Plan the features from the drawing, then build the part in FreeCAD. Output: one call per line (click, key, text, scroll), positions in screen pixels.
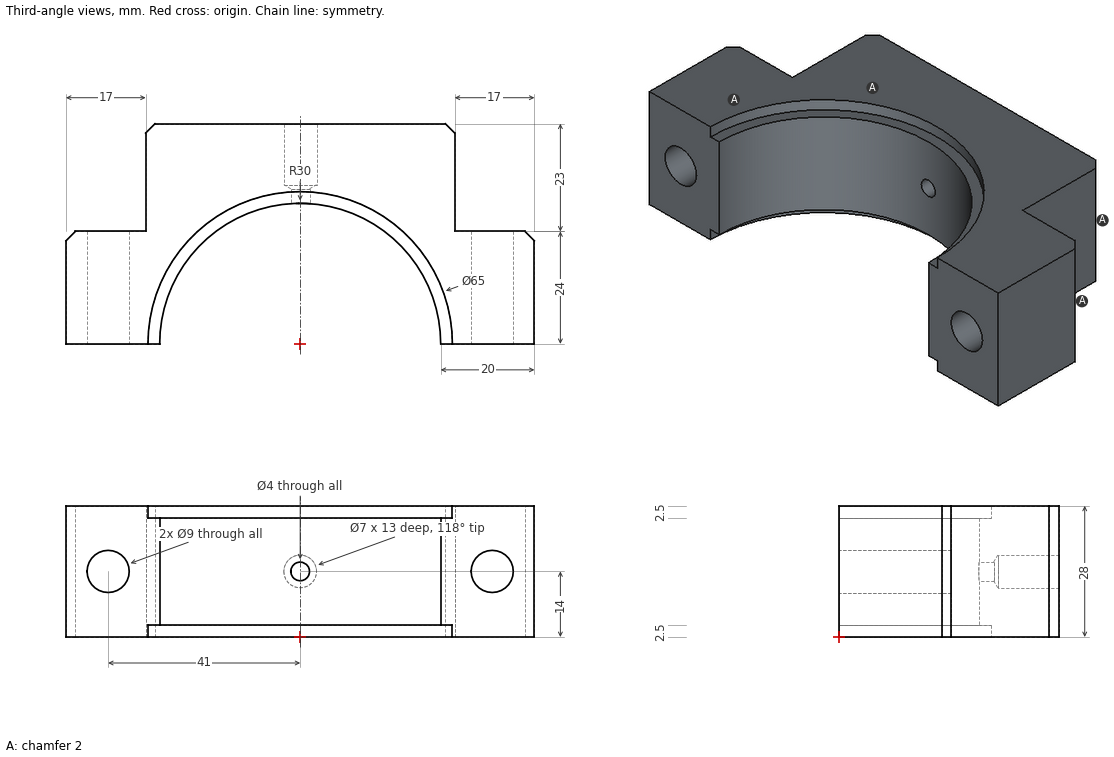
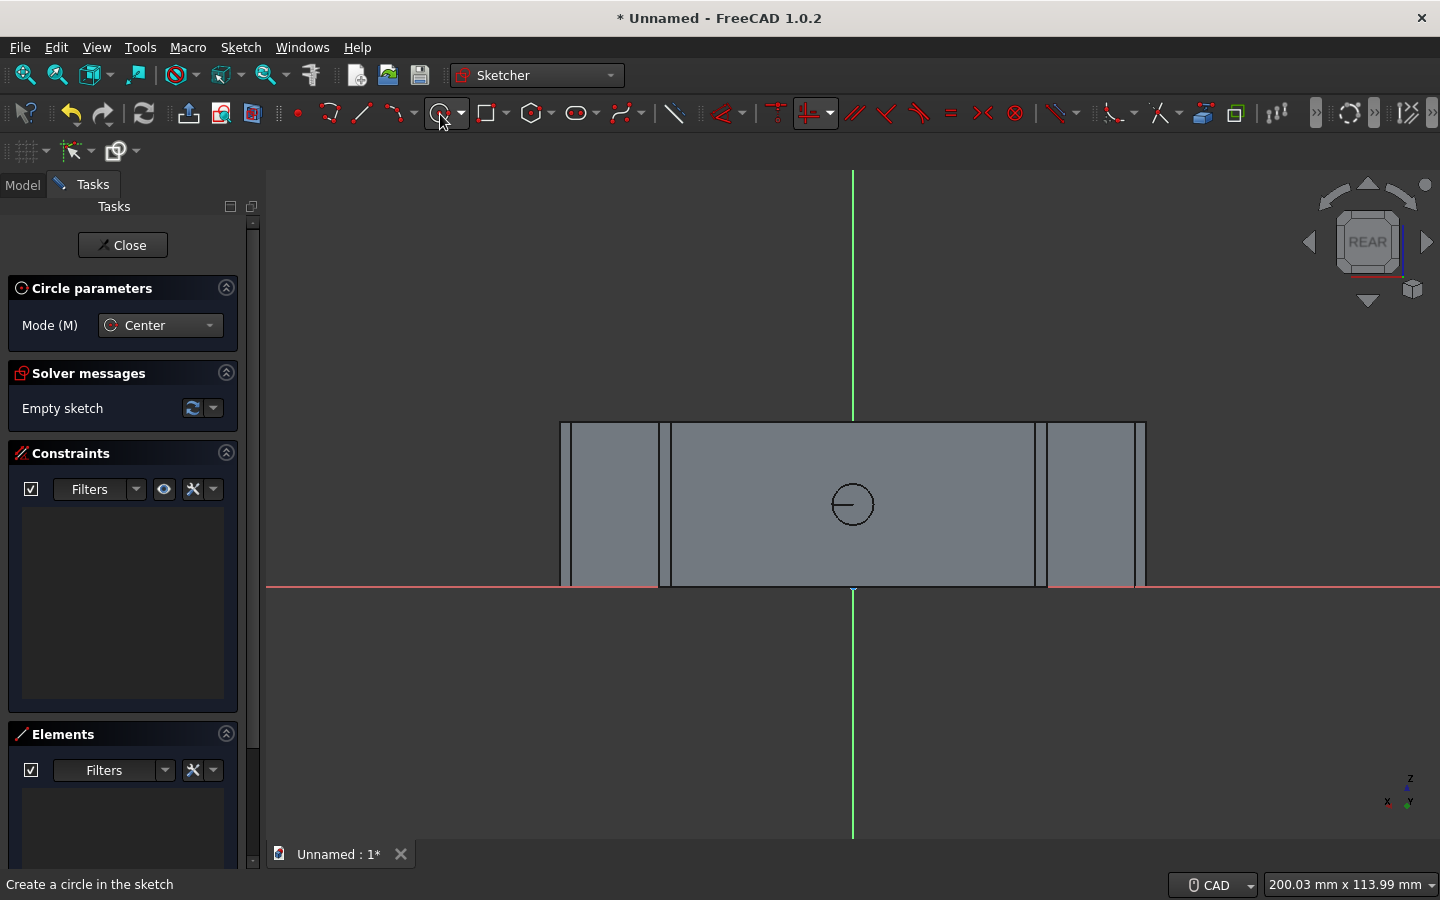
click(1094, 505)
click(1112, 486)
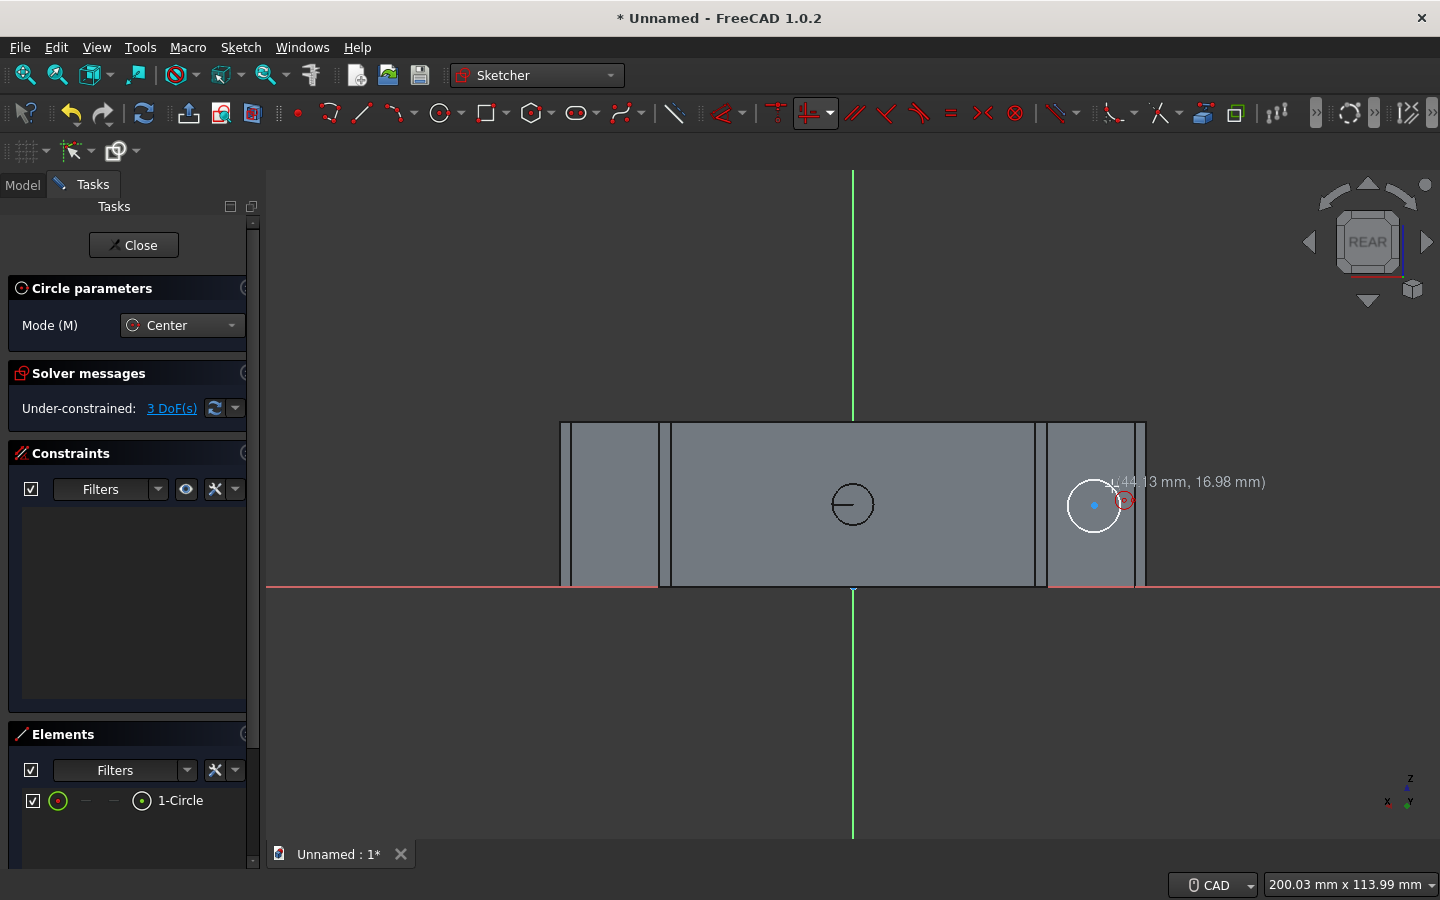
click(612, 505)
click(631, 486)
key(Escape)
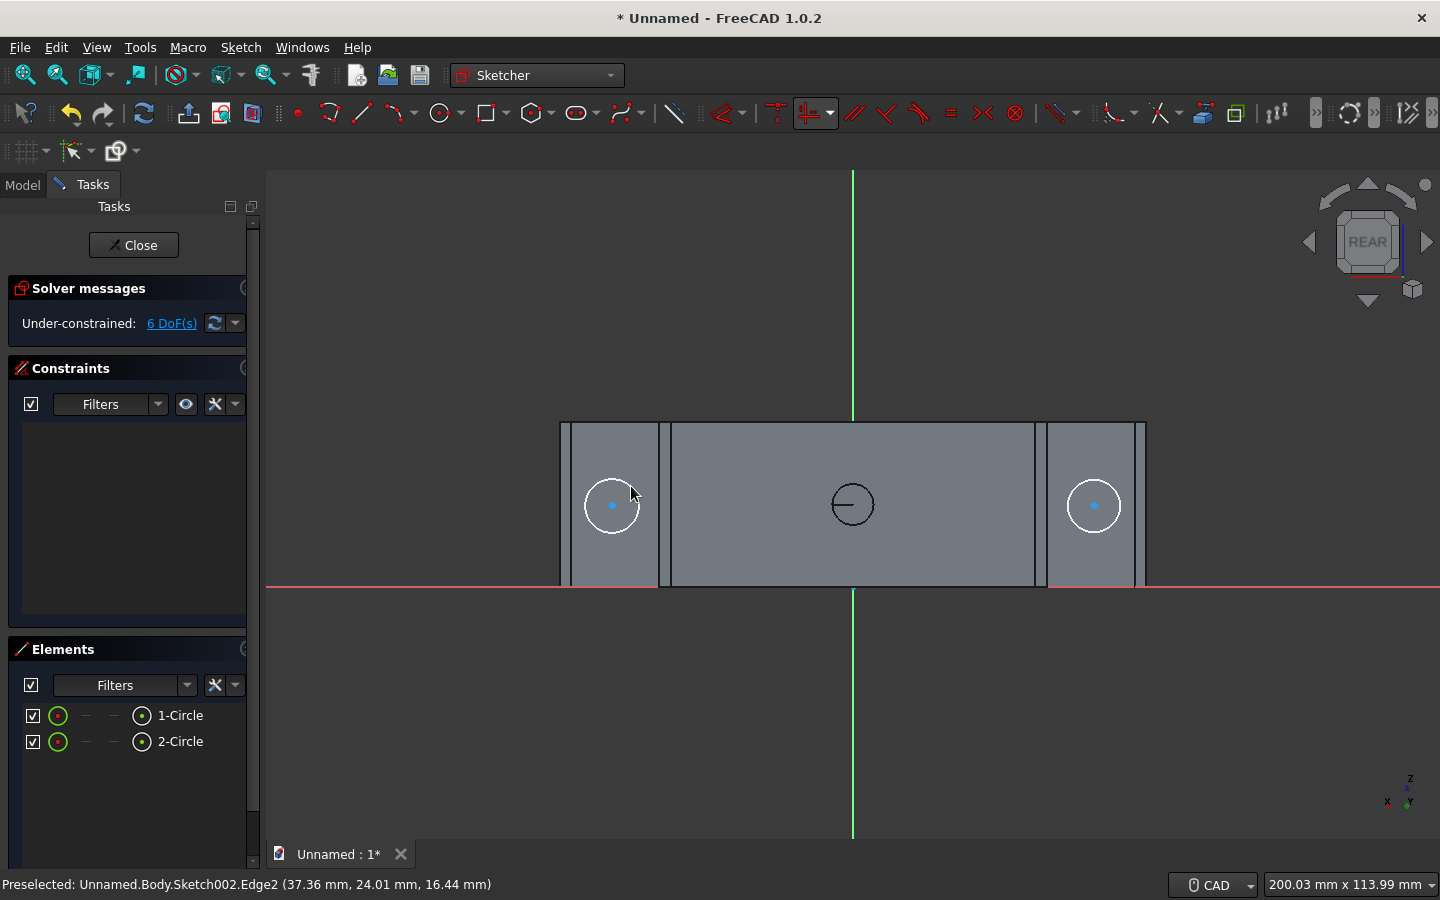
click(1112, 487)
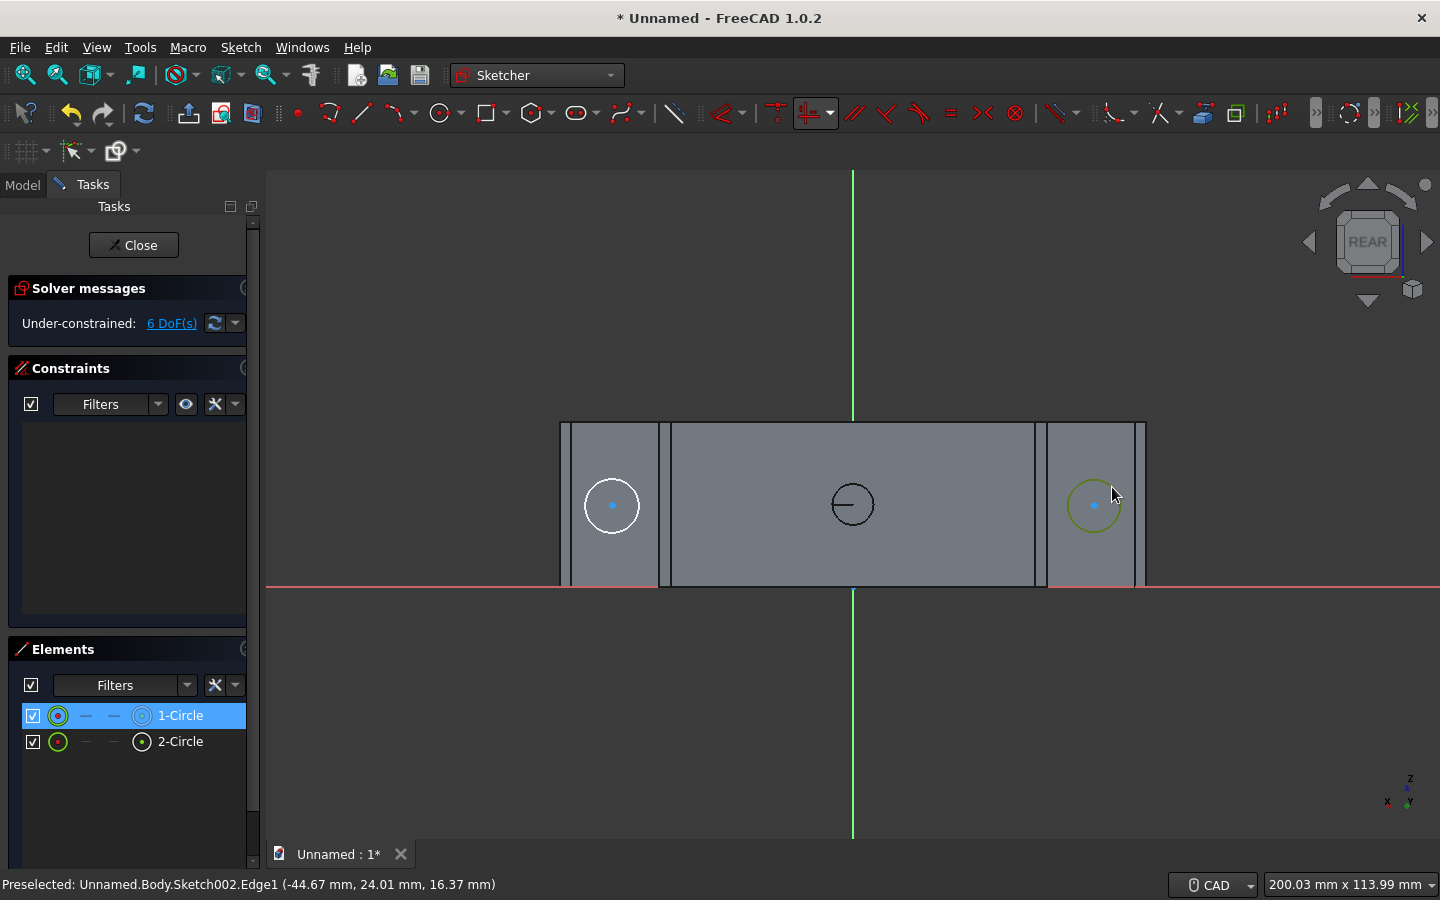
click(631, 487)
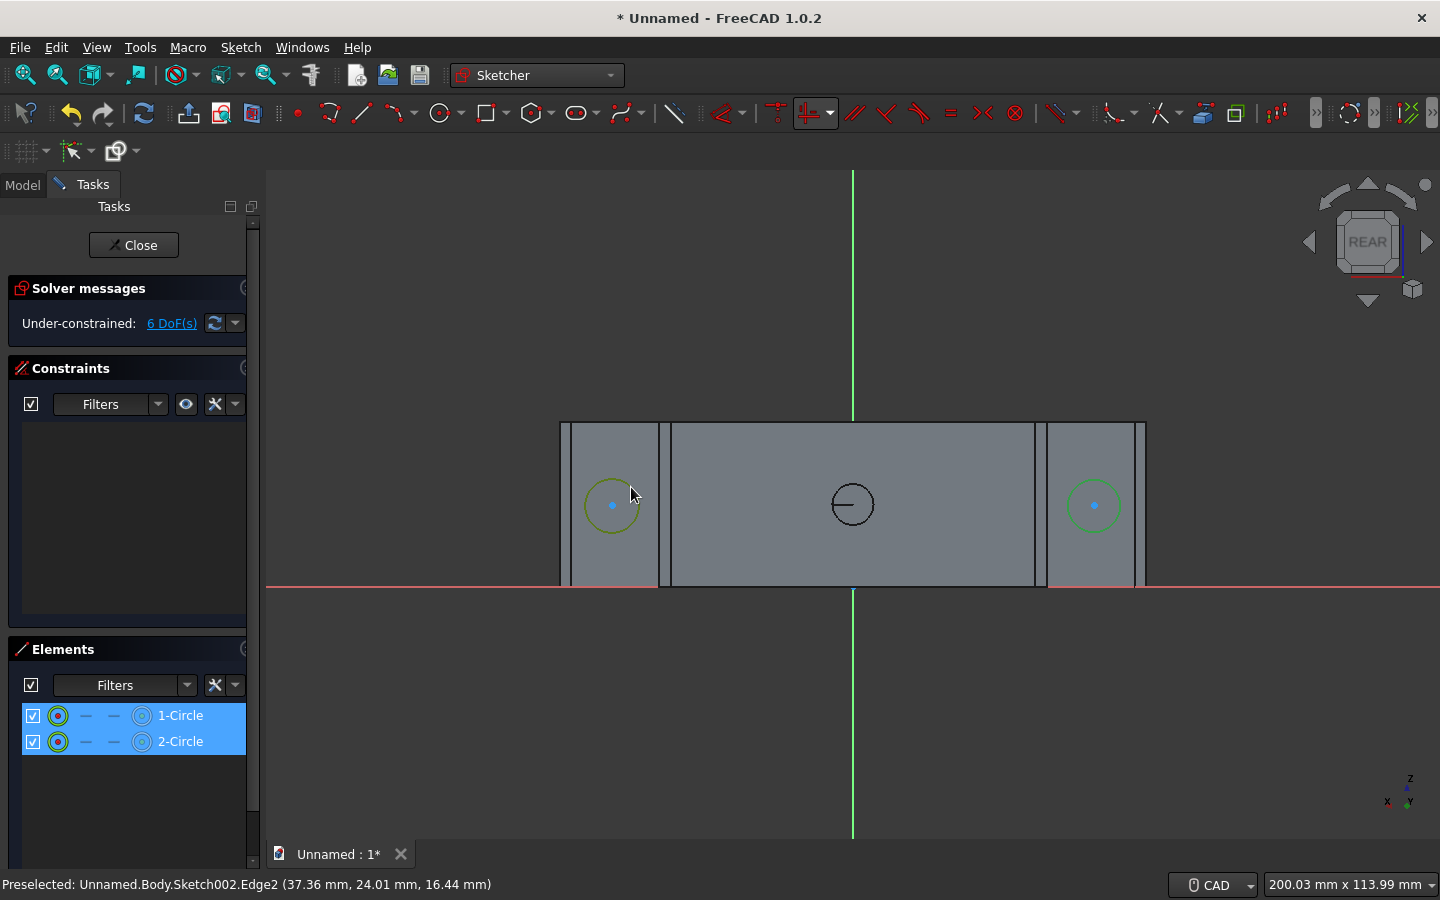
click(952, 114)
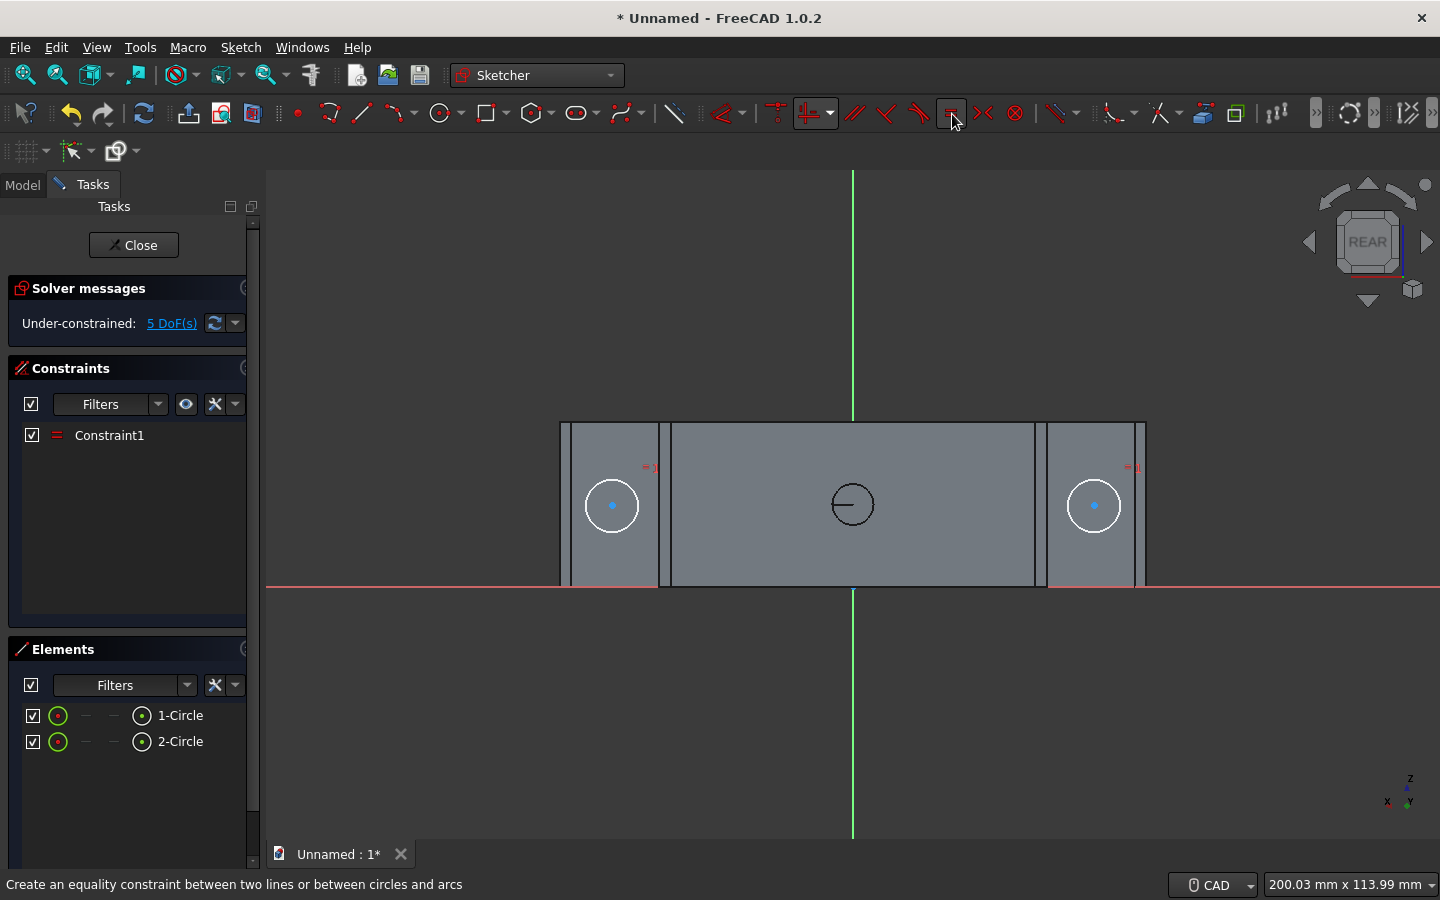
click(1094, 506)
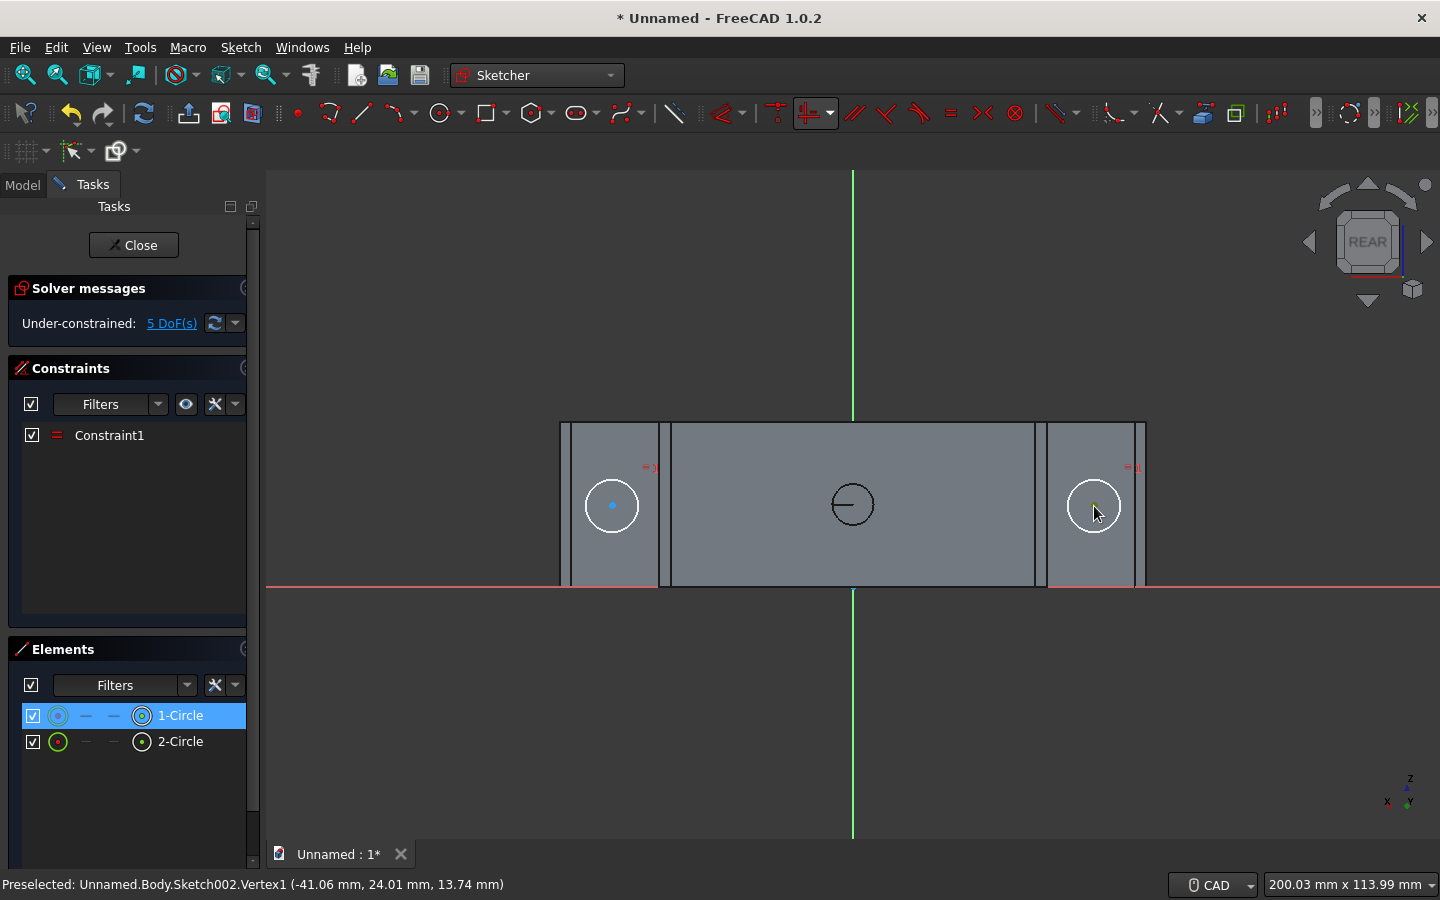
click(612, 506)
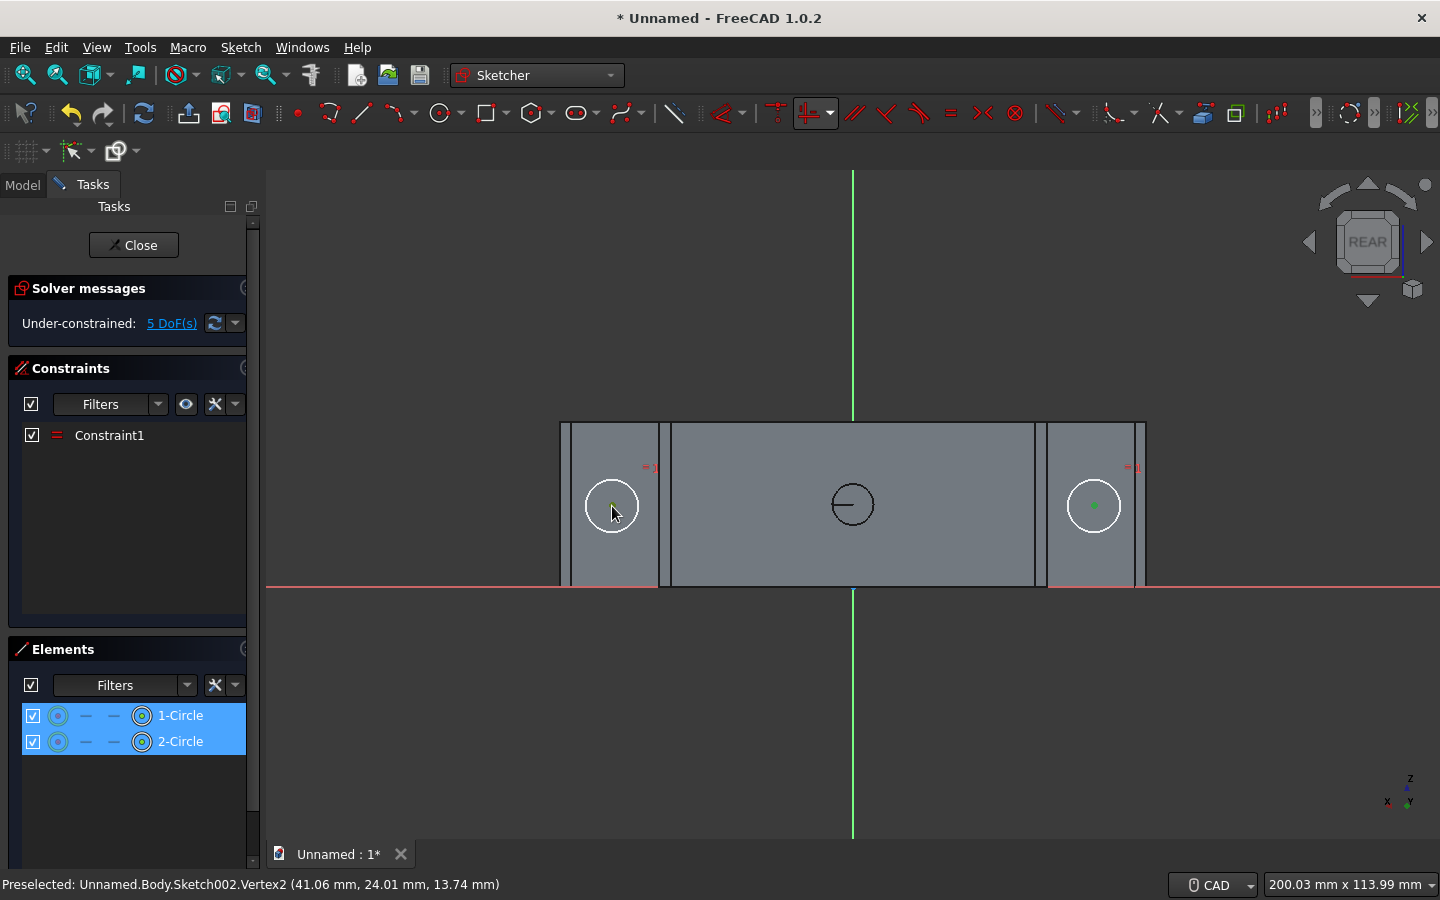
click(853, 767)